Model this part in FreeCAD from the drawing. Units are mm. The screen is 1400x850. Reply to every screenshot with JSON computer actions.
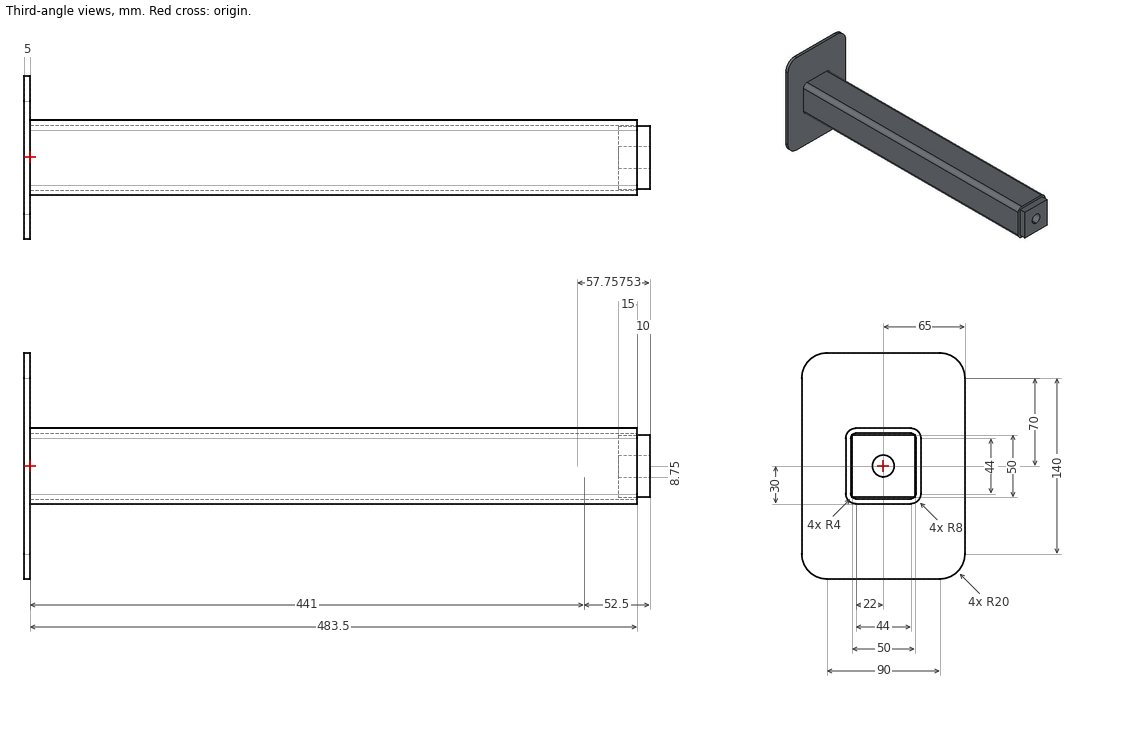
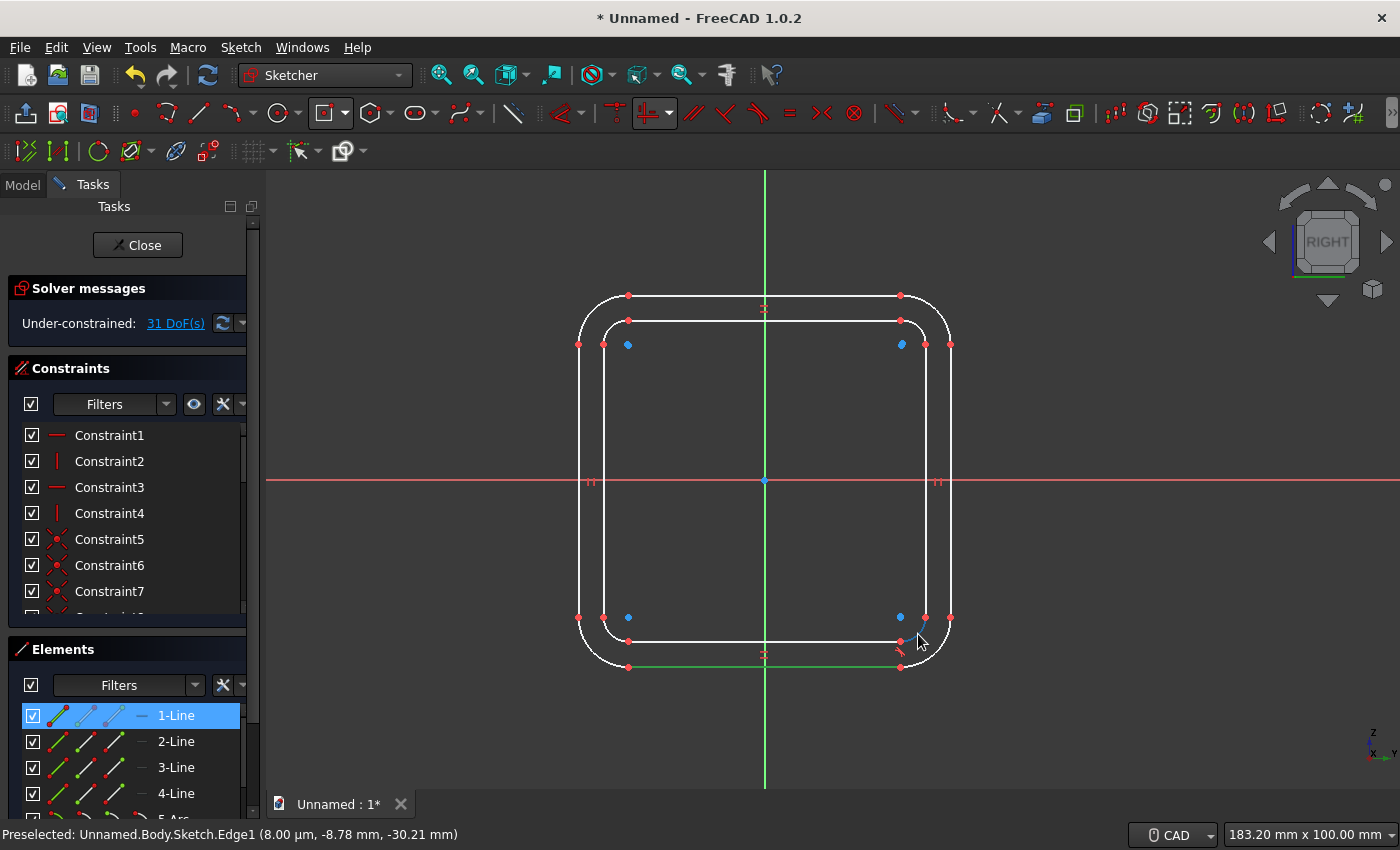
{"action": "left_click", "coordinate": [584, 640]}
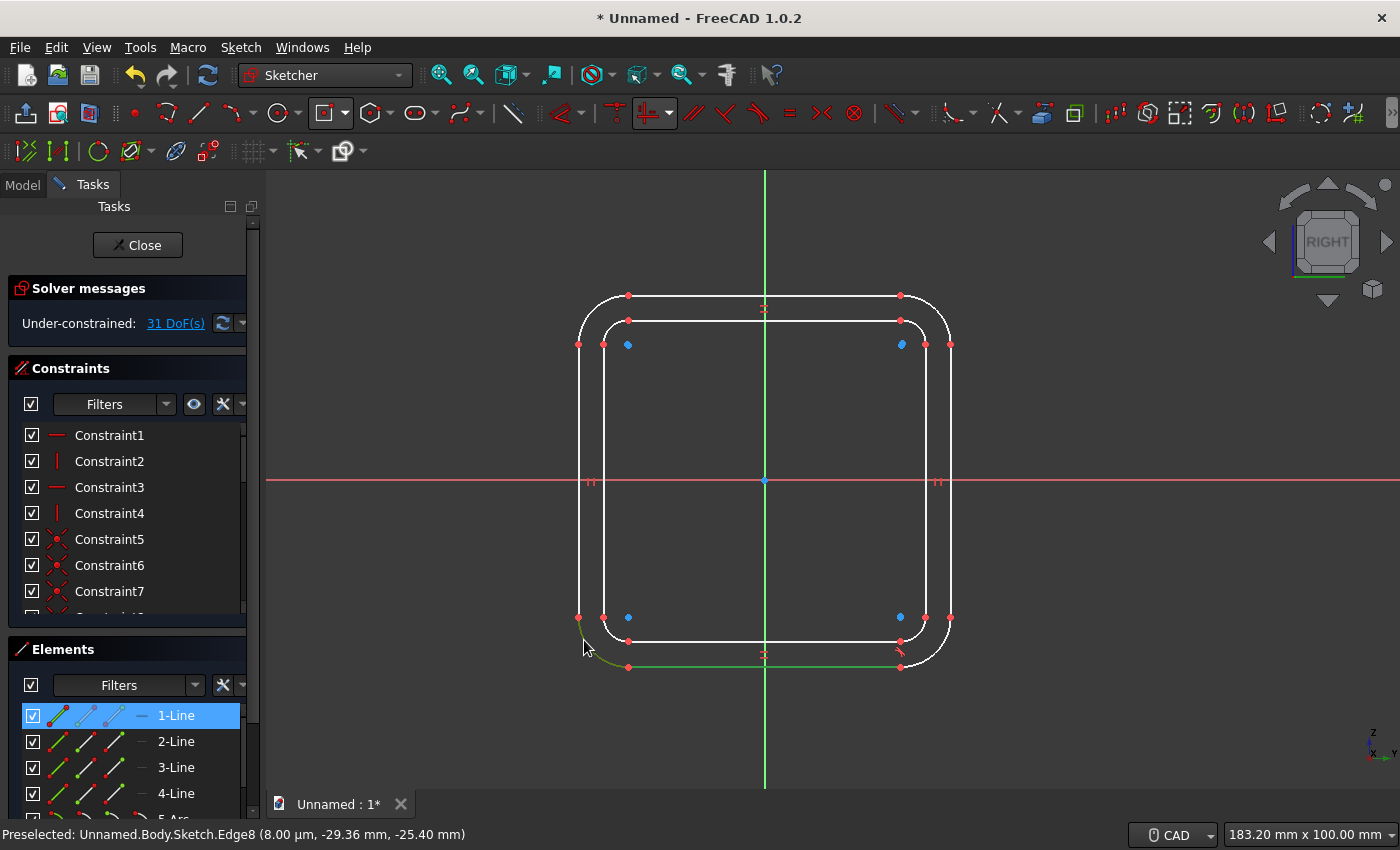
{"action": "key", "text": "t"}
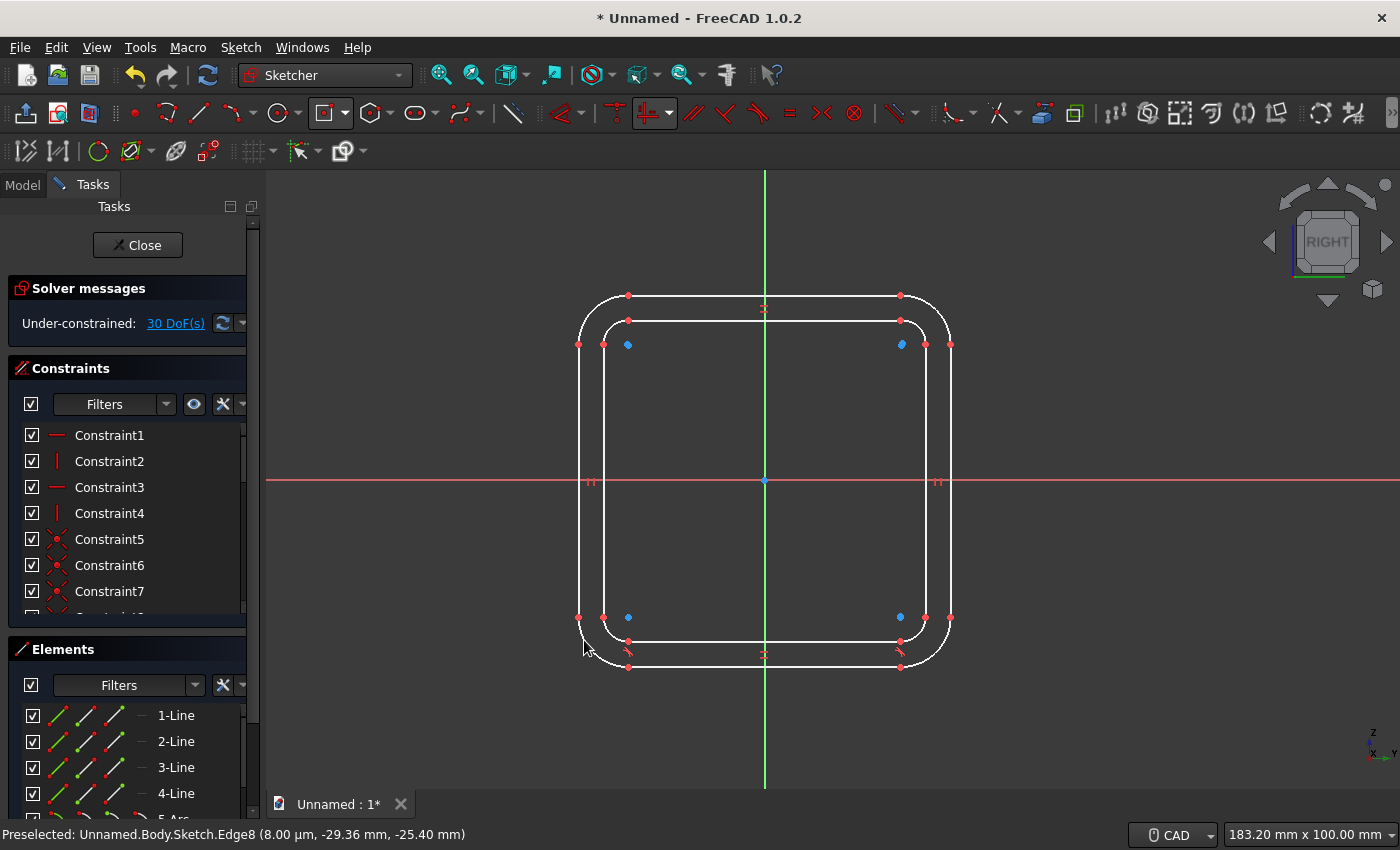
{"action": "left_click", "coordinate": [951, 536]}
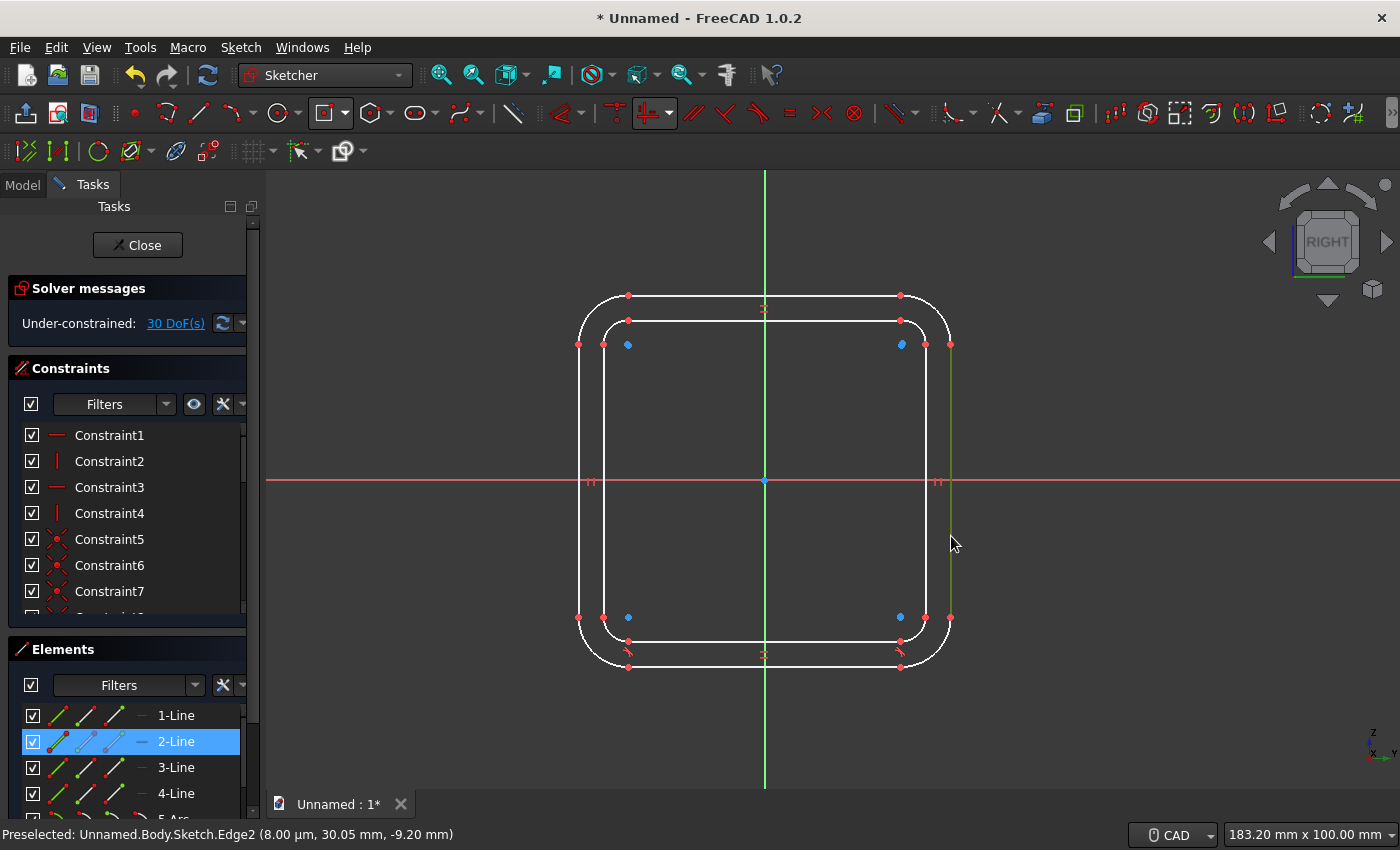
{"action": "left_click", "coordinate": [923, 662]}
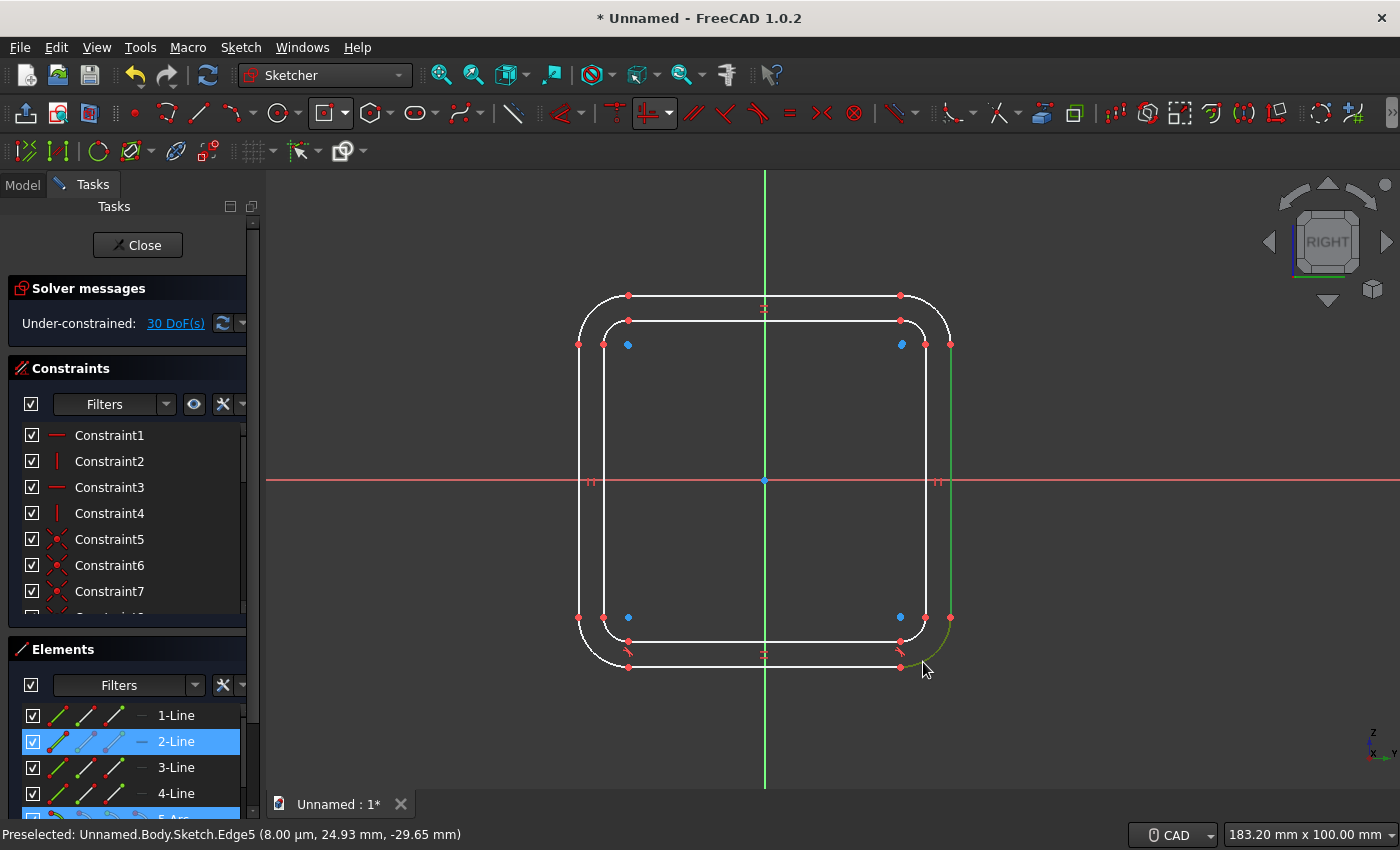
{"action": "left_click", "coordinate": [758, 114]}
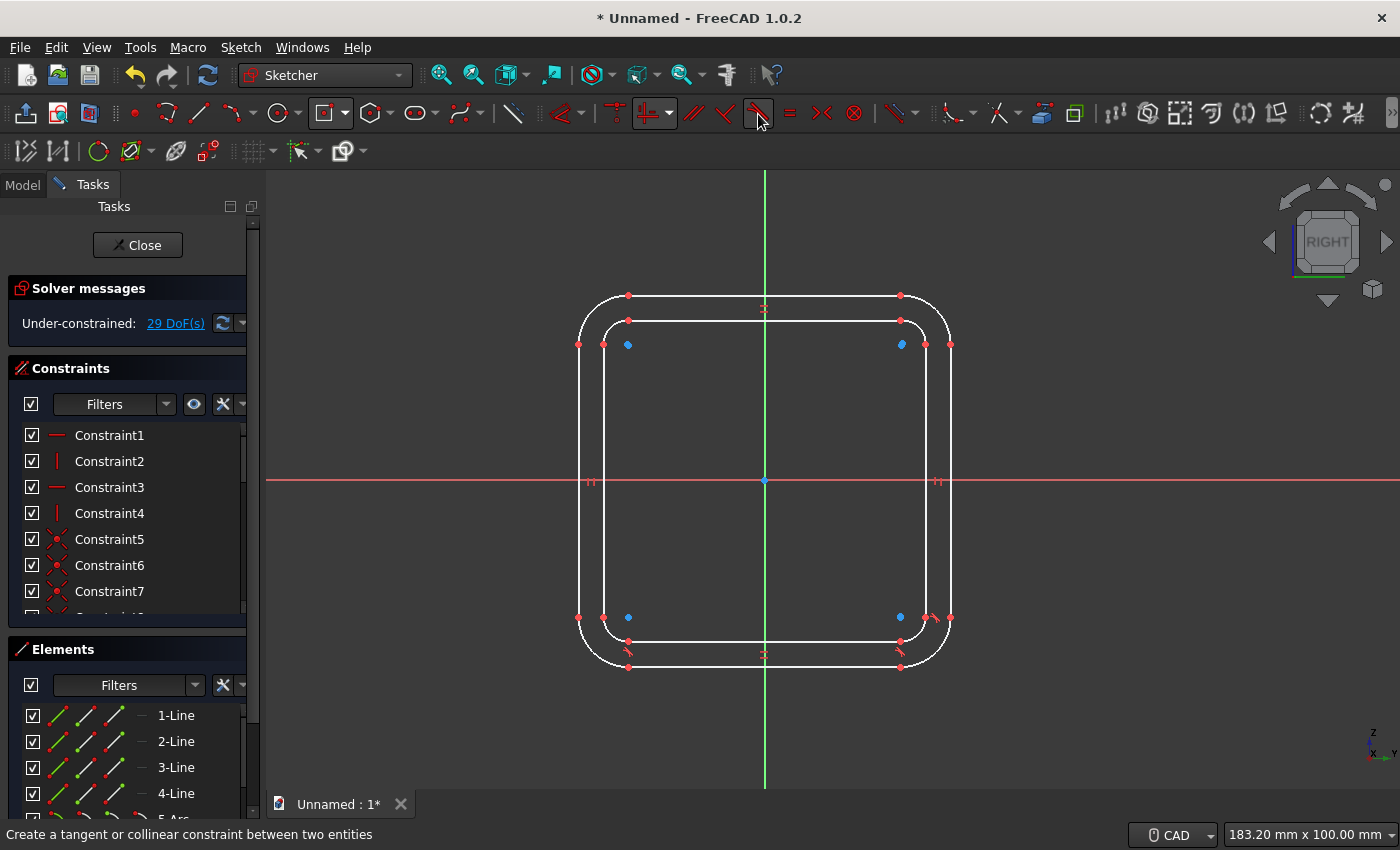
{"action": "left_click", "coordinate": [951, 535]}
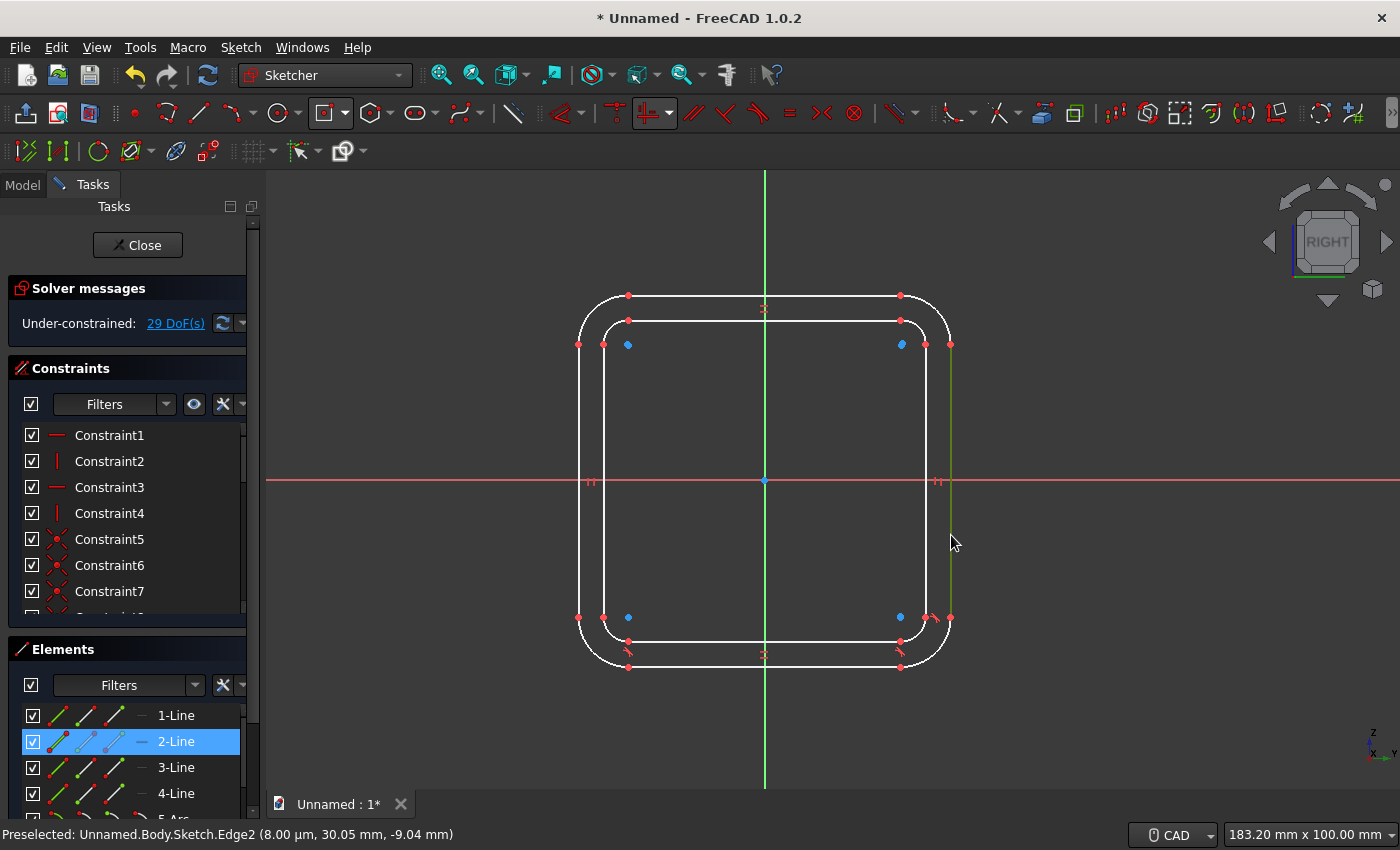
{"action": "left_click", "coordinate": [945, 322]}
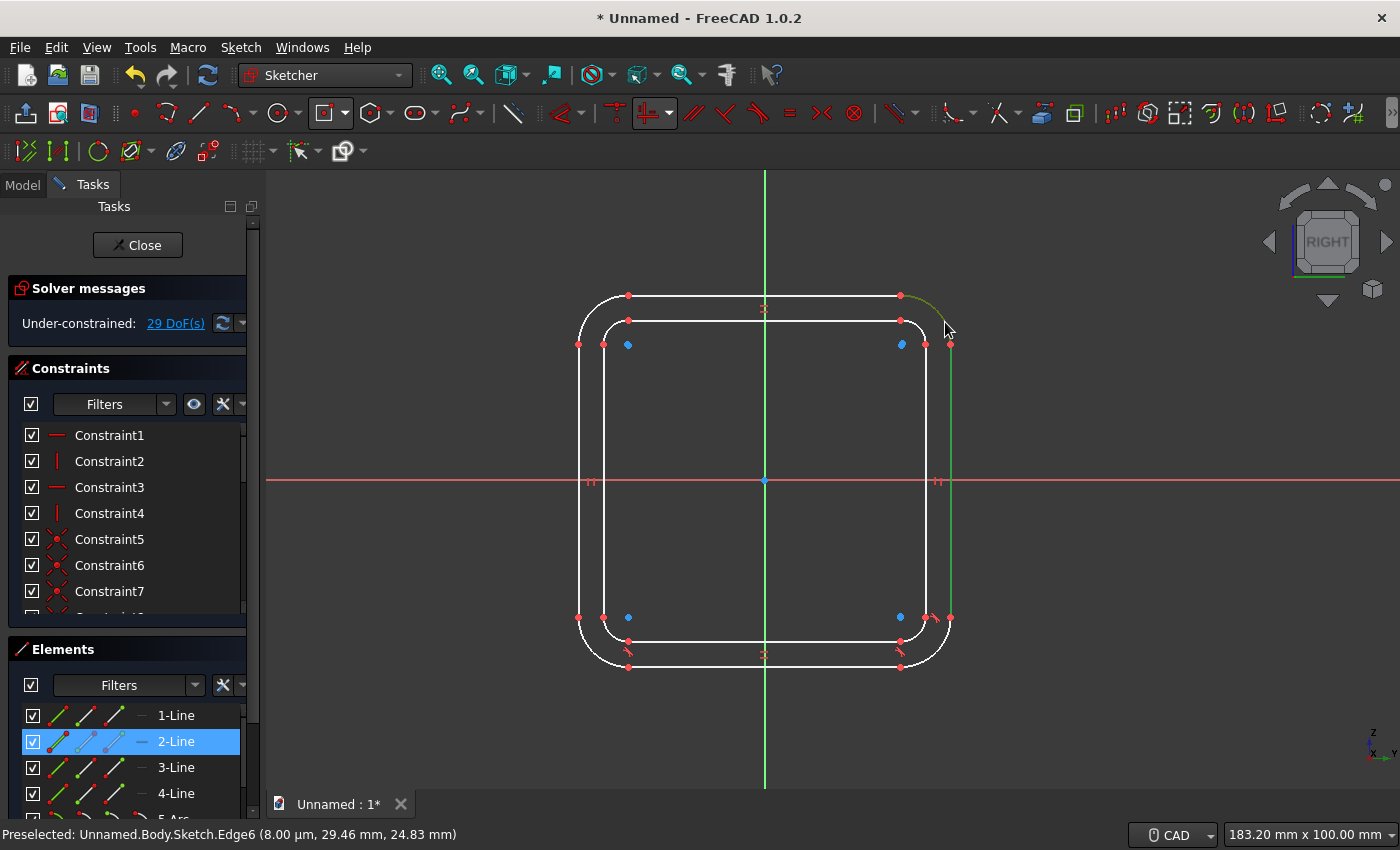
{"action": "left_click", "coordinate": [758, 114]}